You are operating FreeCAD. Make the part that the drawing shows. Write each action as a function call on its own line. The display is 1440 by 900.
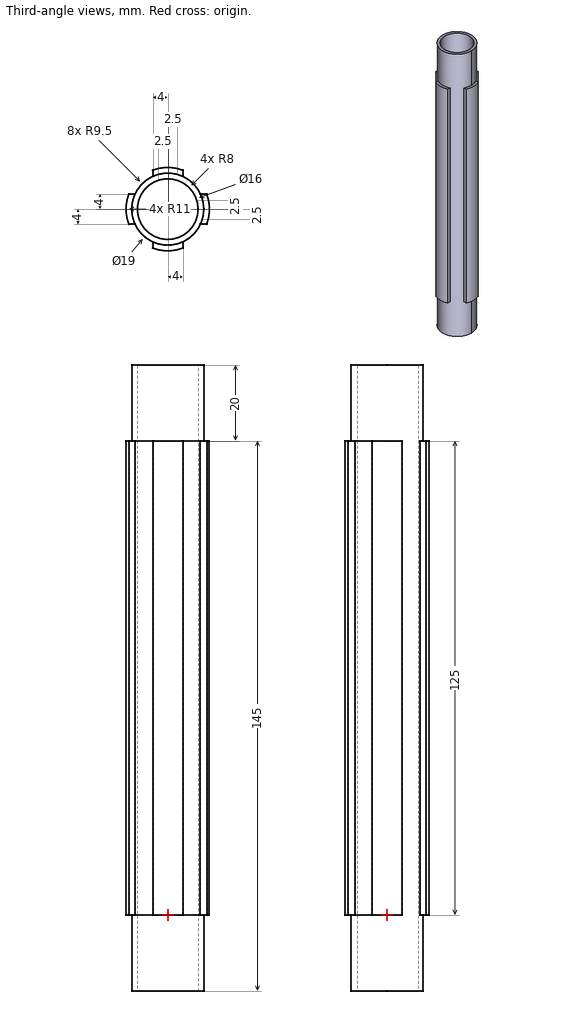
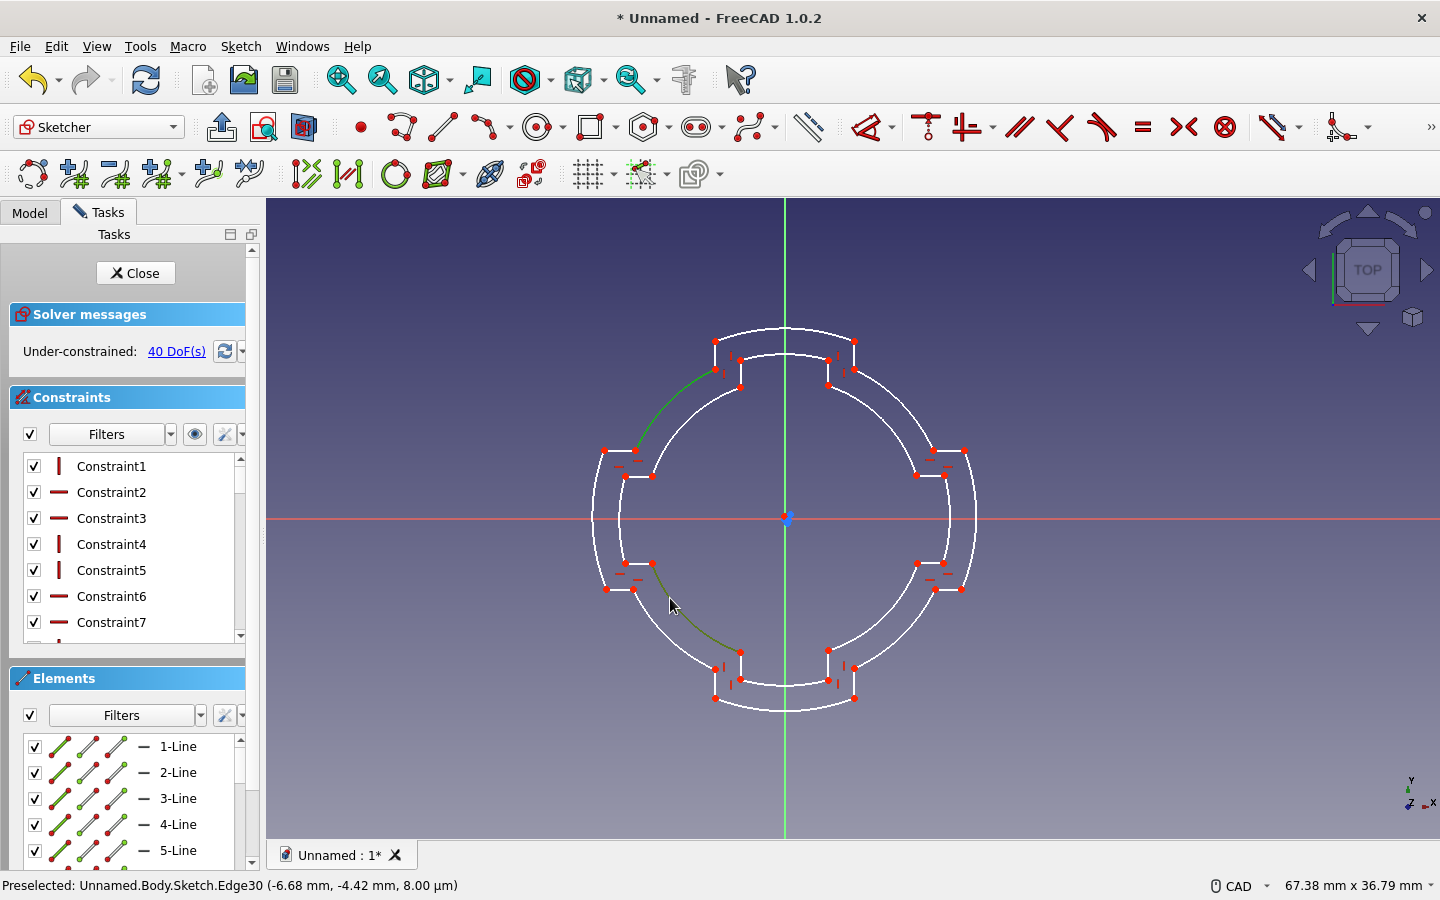
click(926, 128)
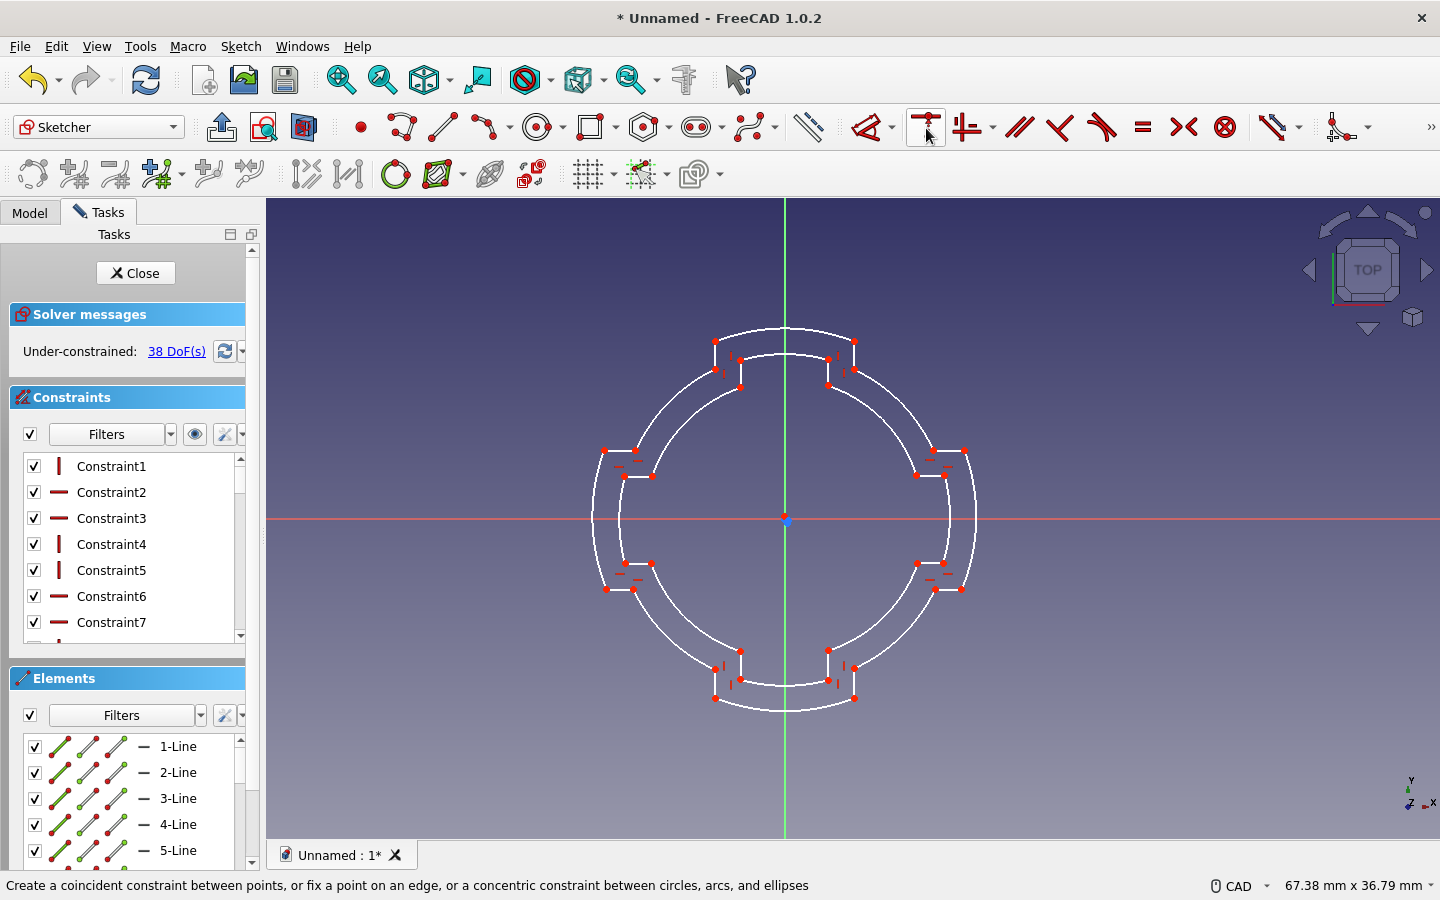
click(686, 387)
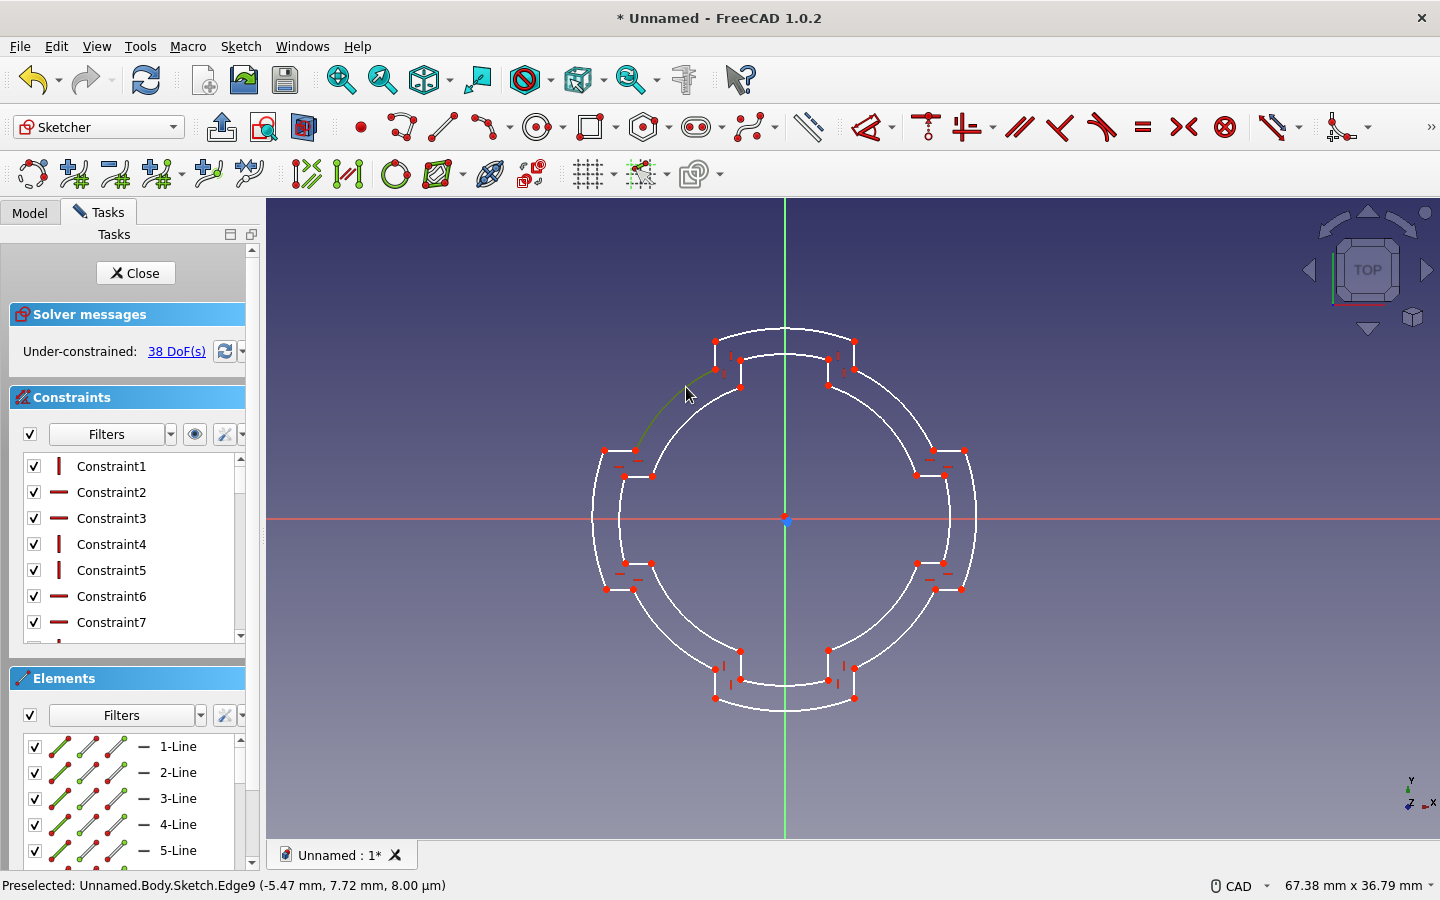
click(620, 503)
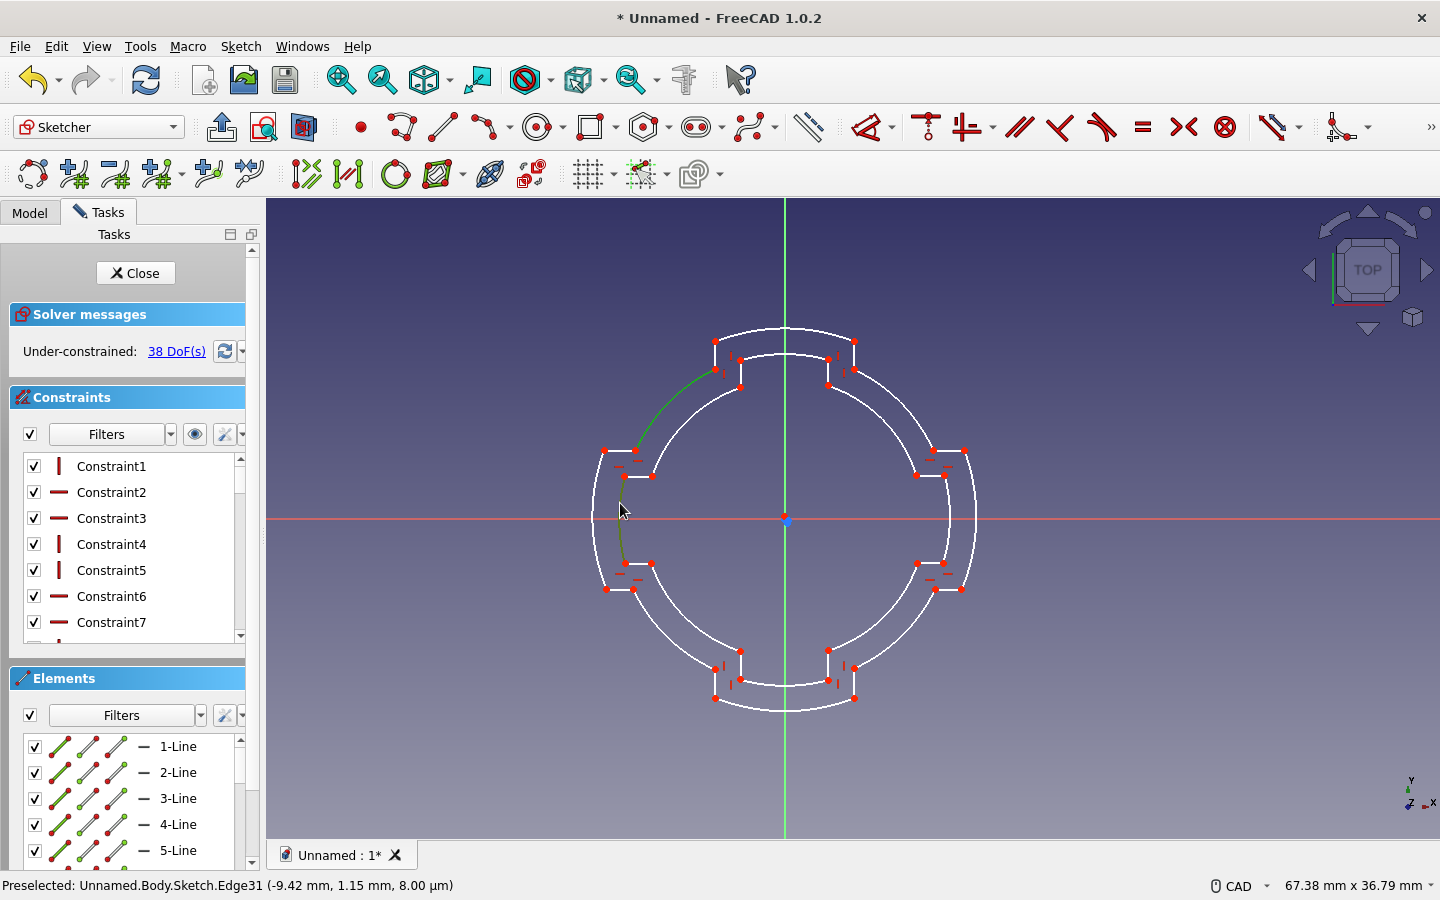
click(926, 128)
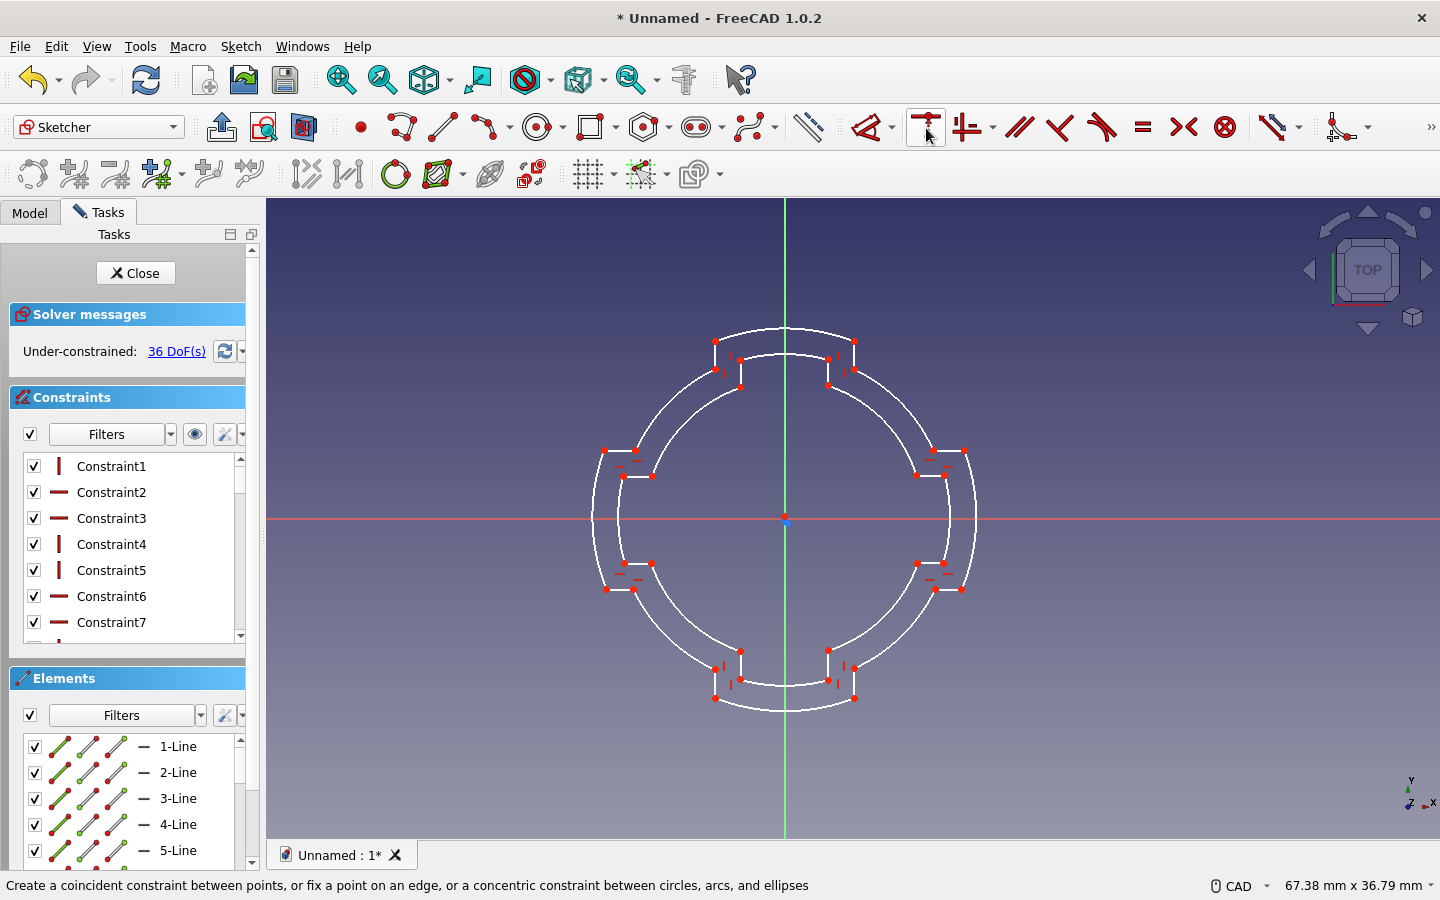
click(686, 387)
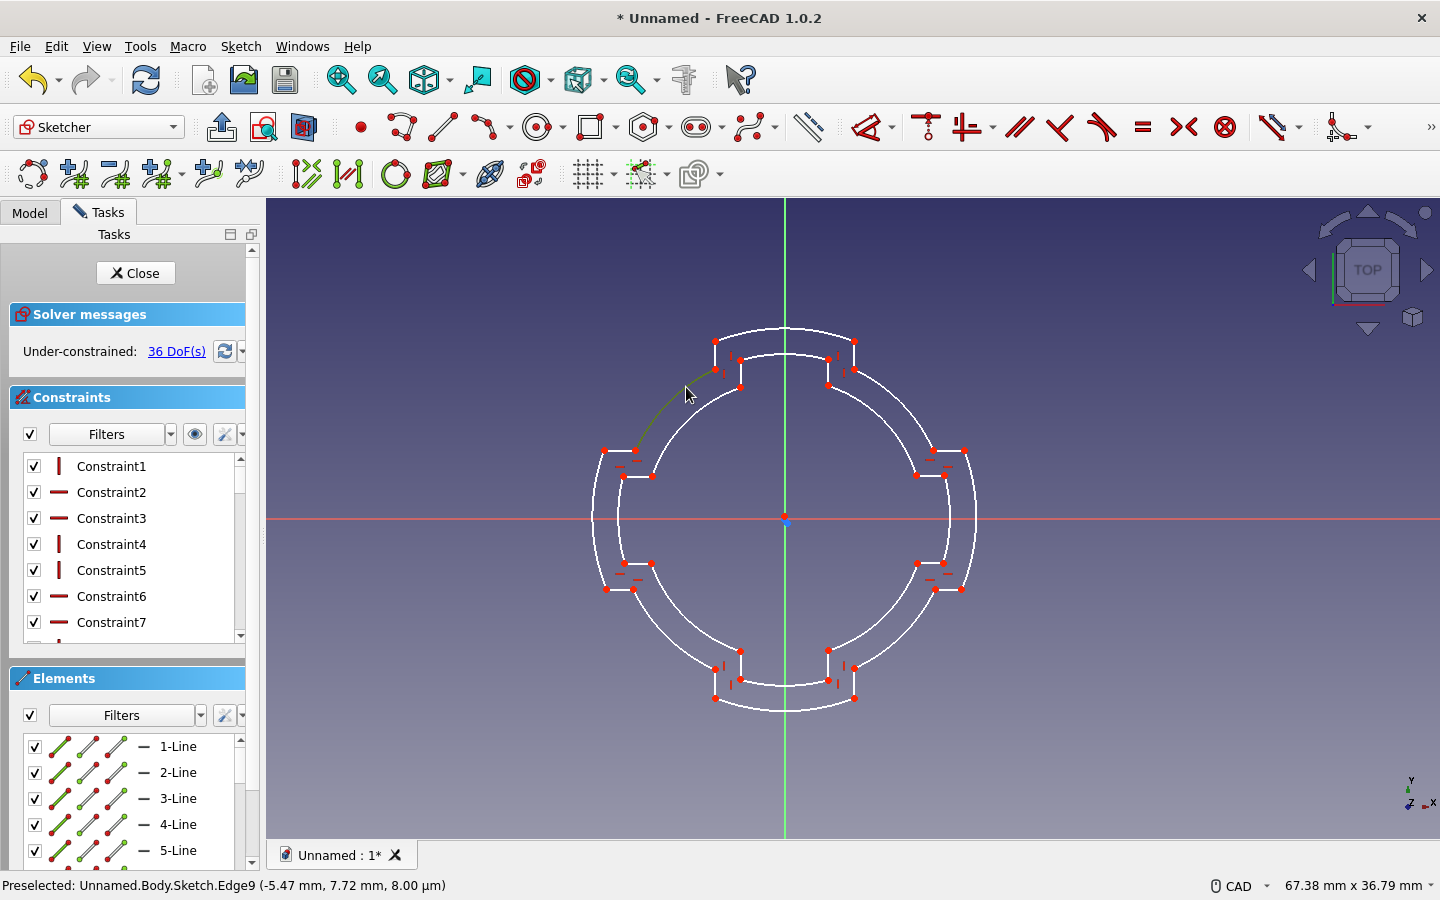
click(706, 405)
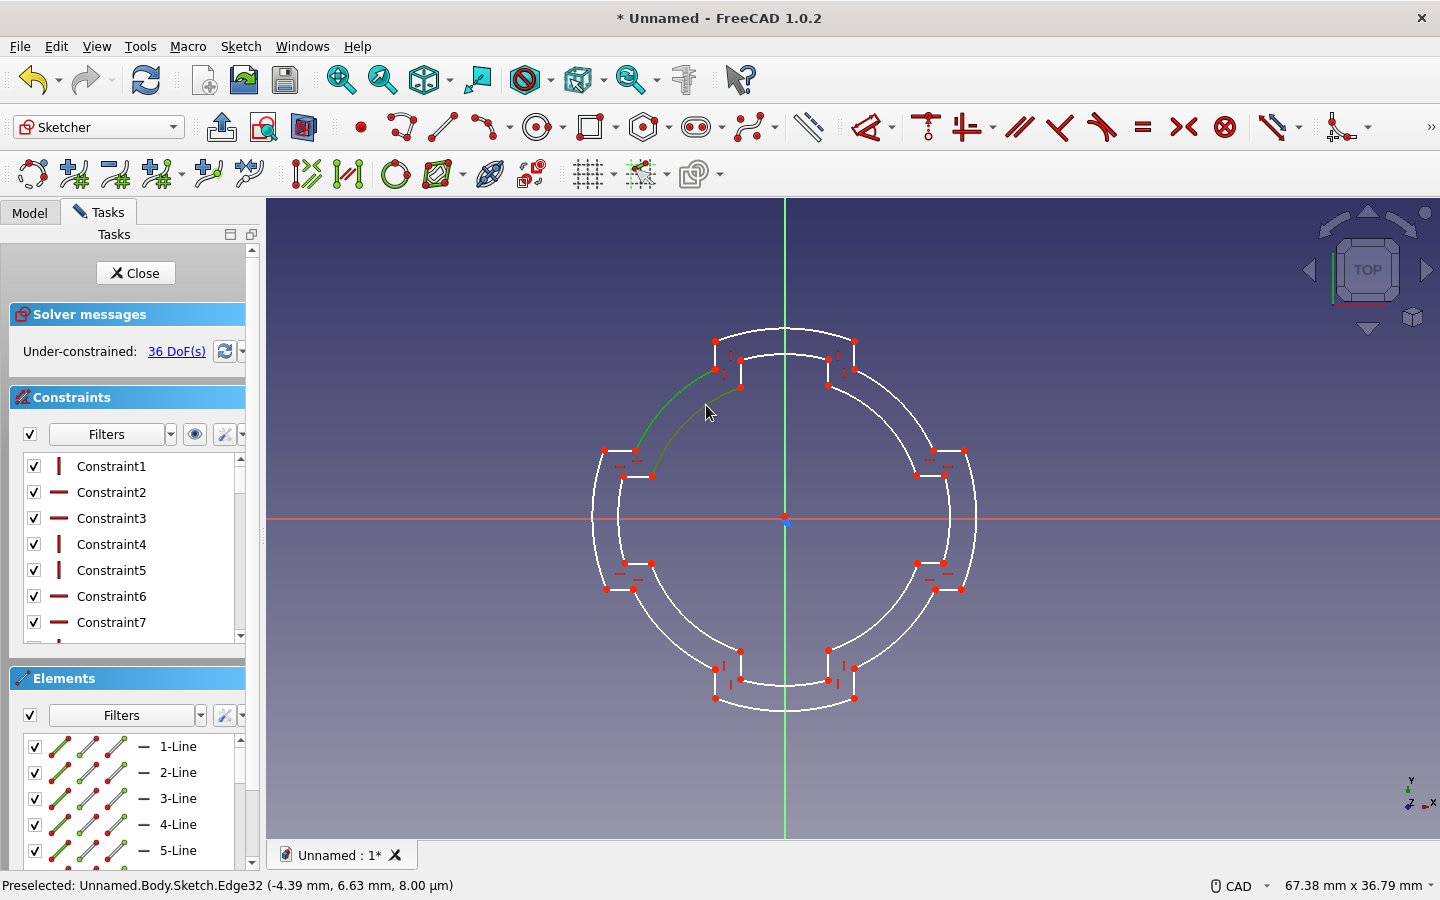
click(926, 128)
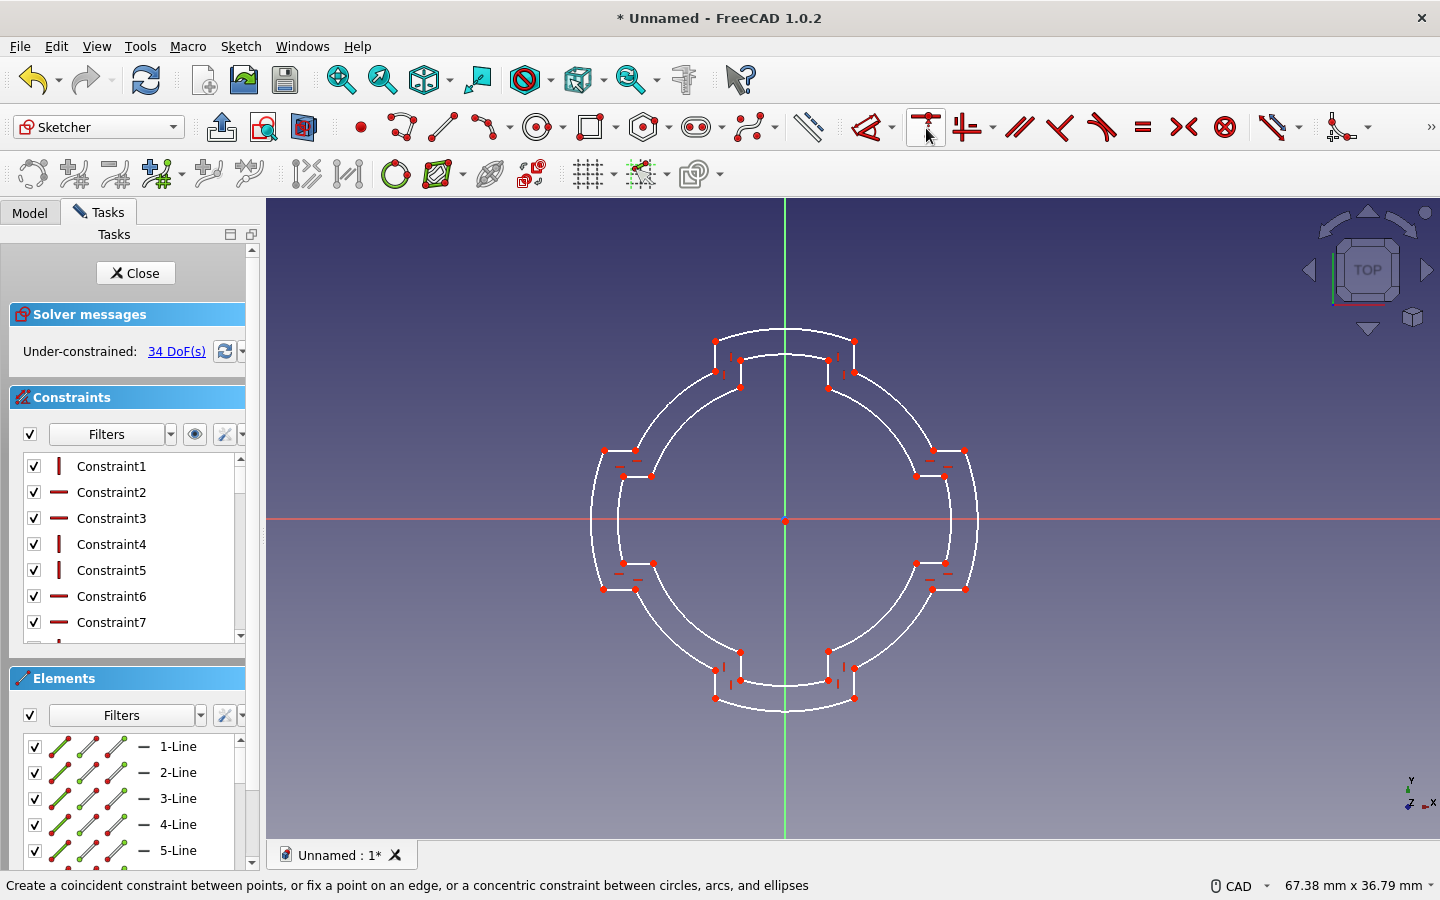
drag(775, 509, 795, 531)